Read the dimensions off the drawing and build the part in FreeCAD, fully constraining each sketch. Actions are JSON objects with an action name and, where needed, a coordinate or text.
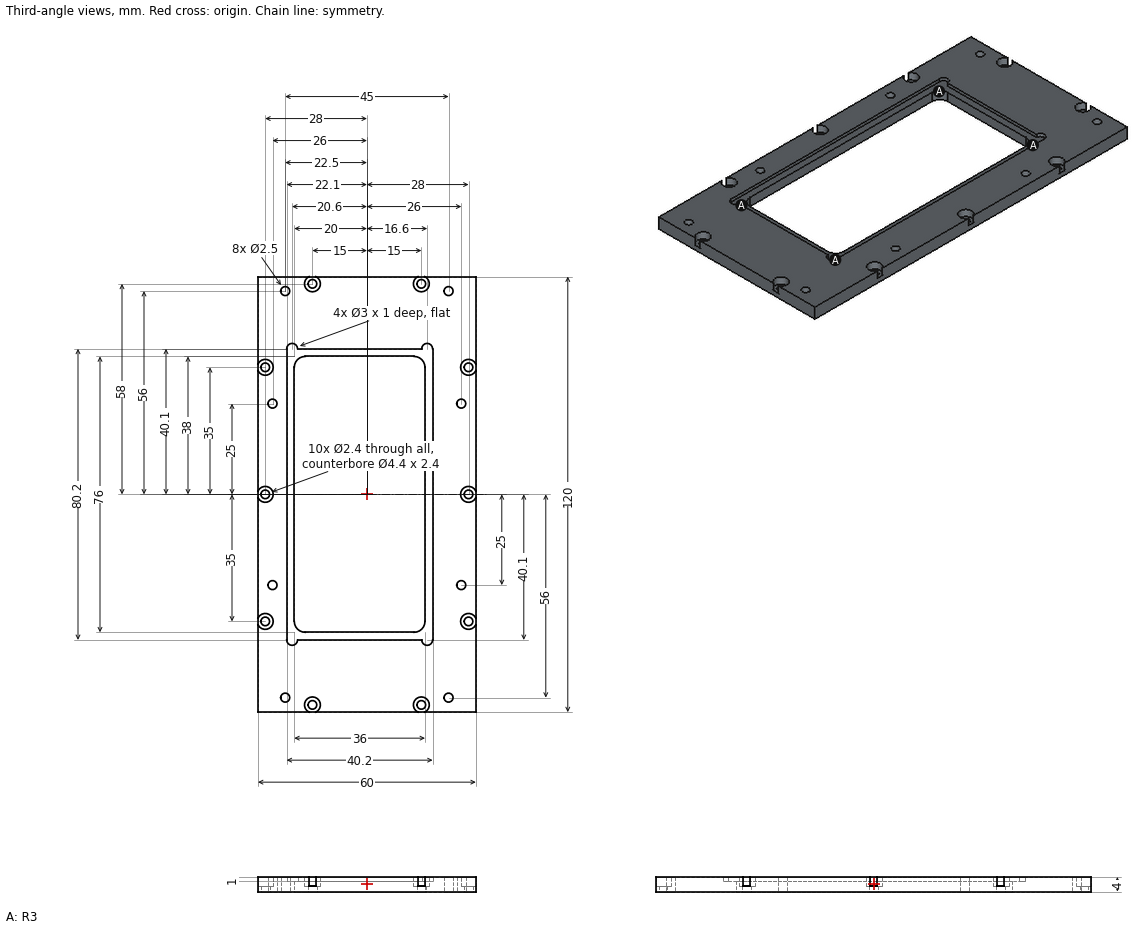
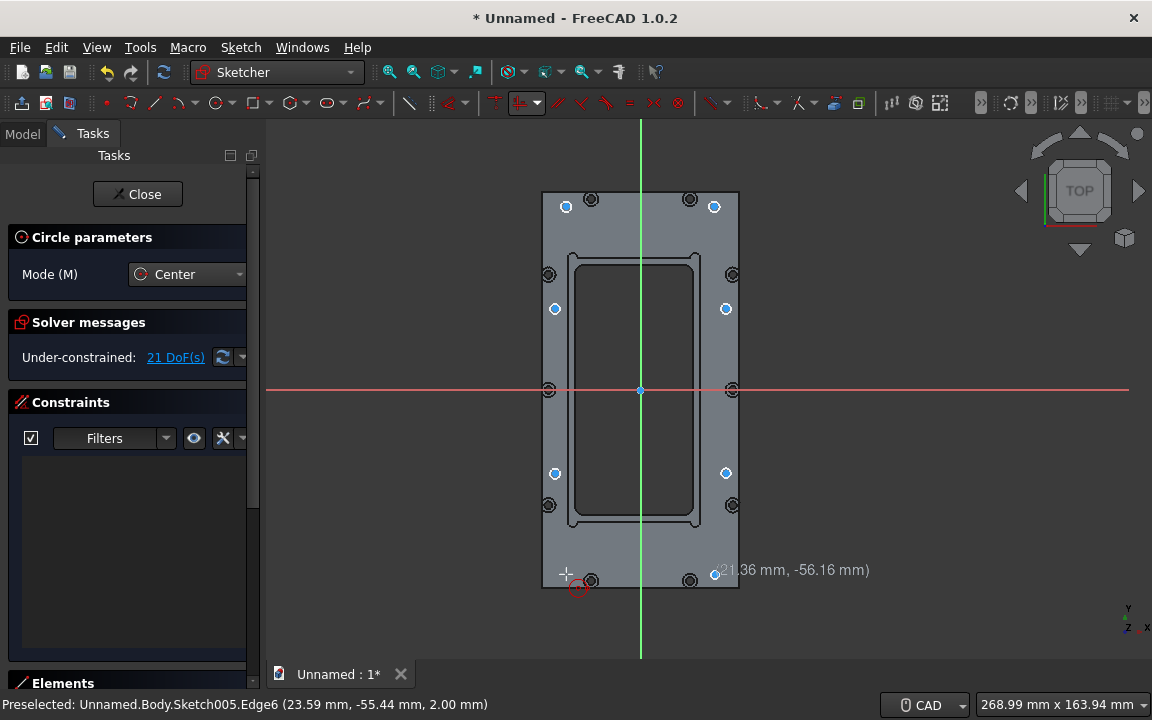
{"action": "left_click", "coordinate": [566, 574]}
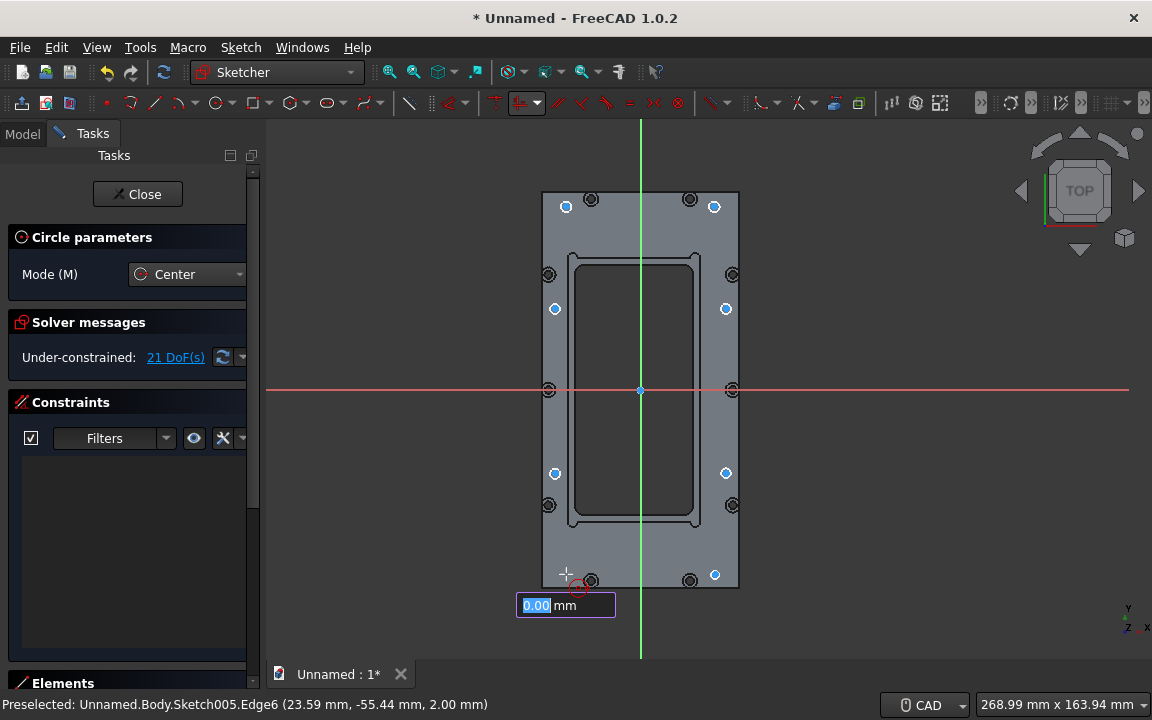
{"action": "scroll", "coordinate": [569, 572], "scroll_direction": "up", "scroll_amount": 7}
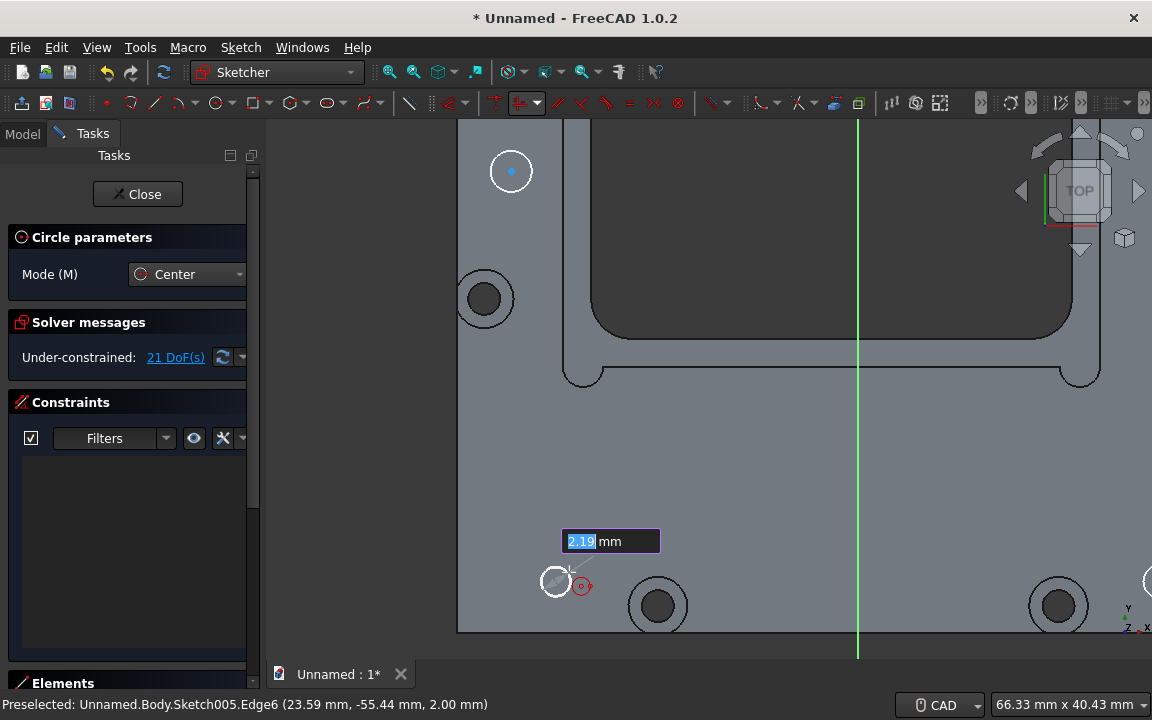
{"action": "left_click", "coordinate": [569, 568]}
{"action": "key", "text": "Escape"}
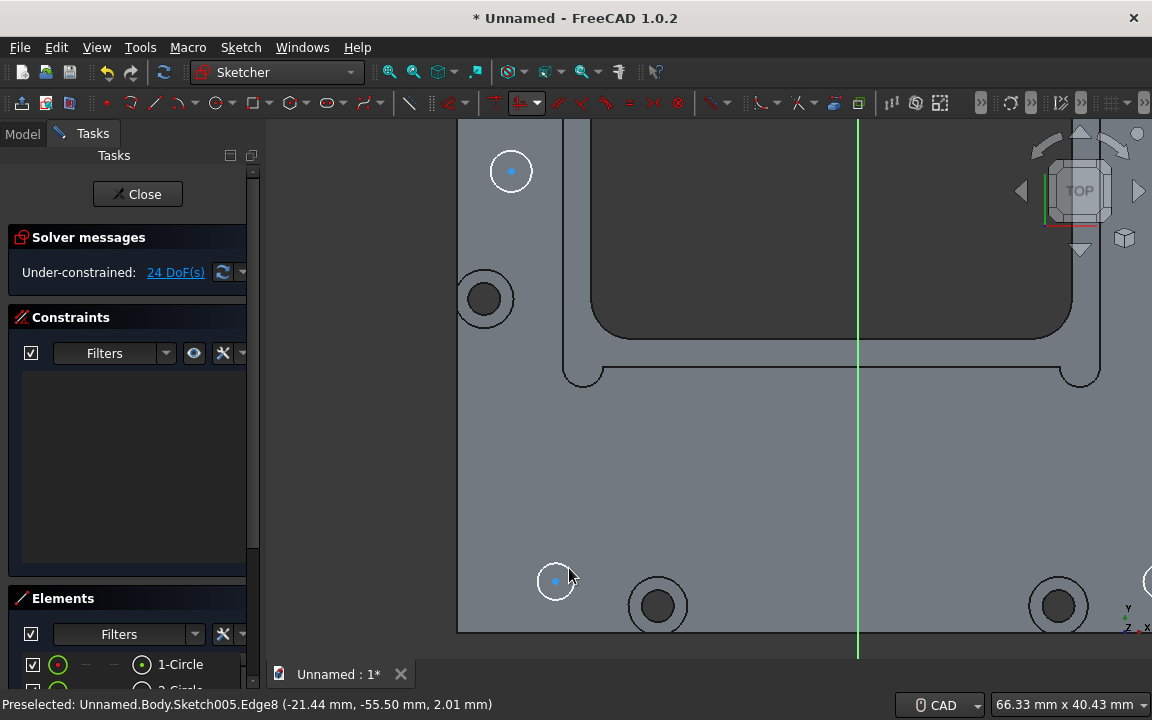
{"action": "scroll", "coordinate": [569, 572], "scroll_direction": "down", "scroll_amount": 7}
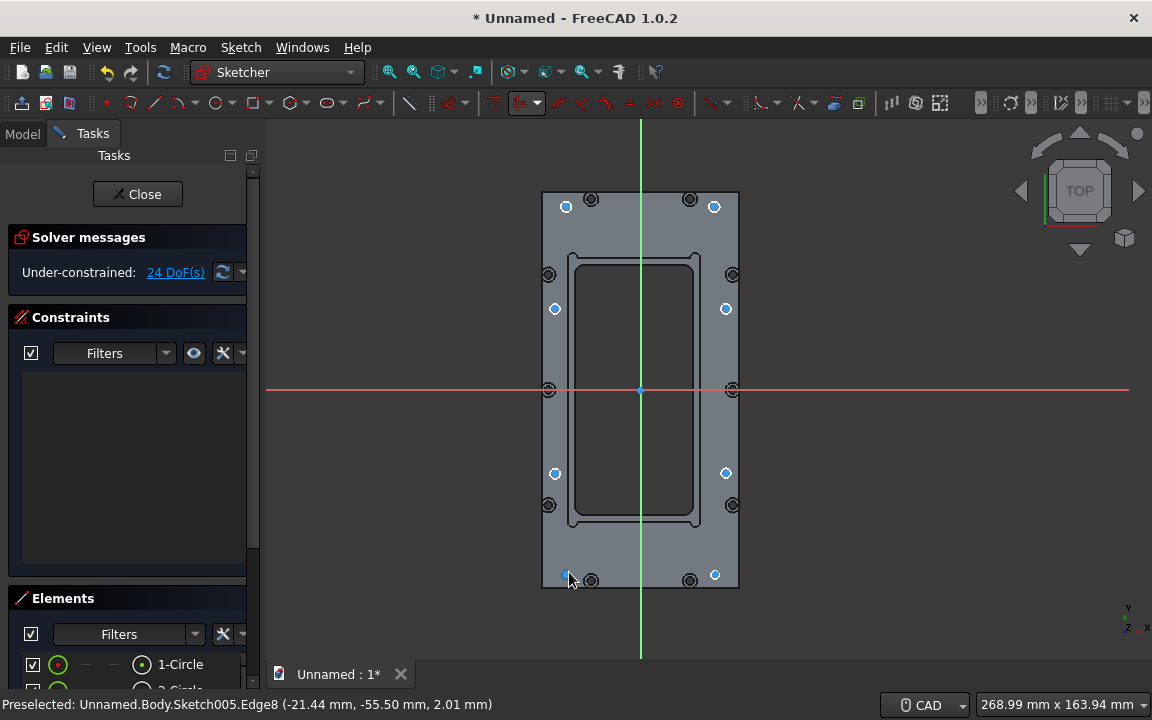
{"action": "scroll", "coordinate": [570, 203], "scroll_direction": "up", "scroll_amount": 5}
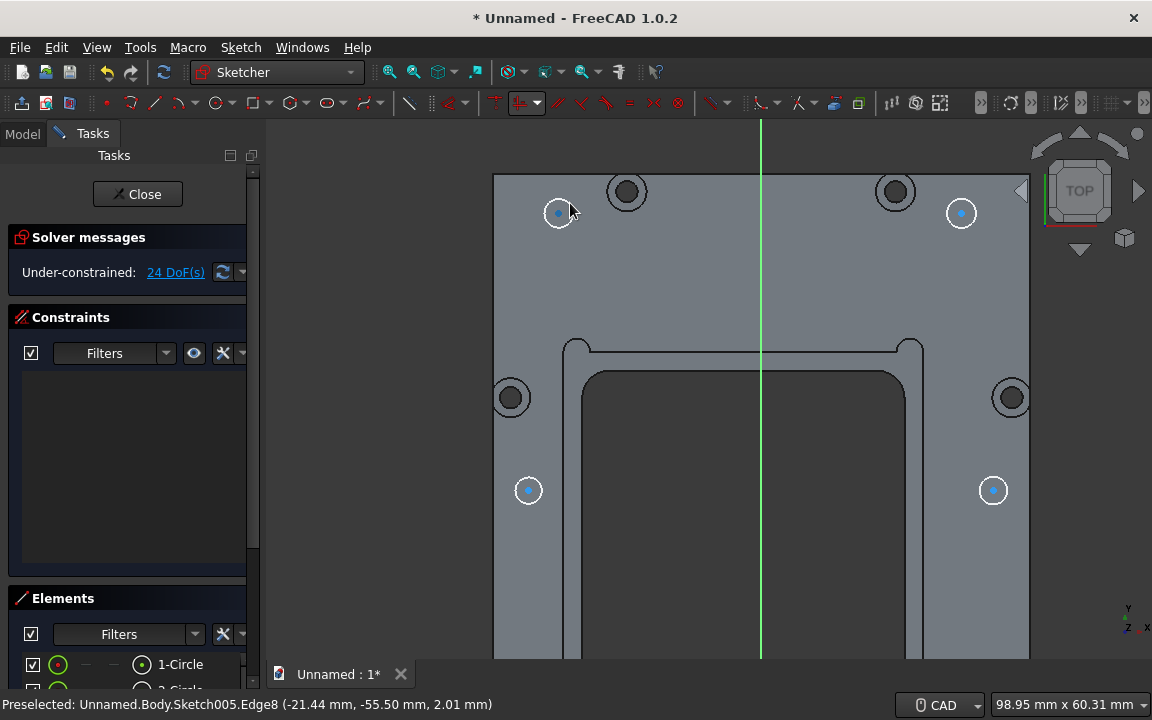
{"action": "left_click", "coordinate": [569, 203]}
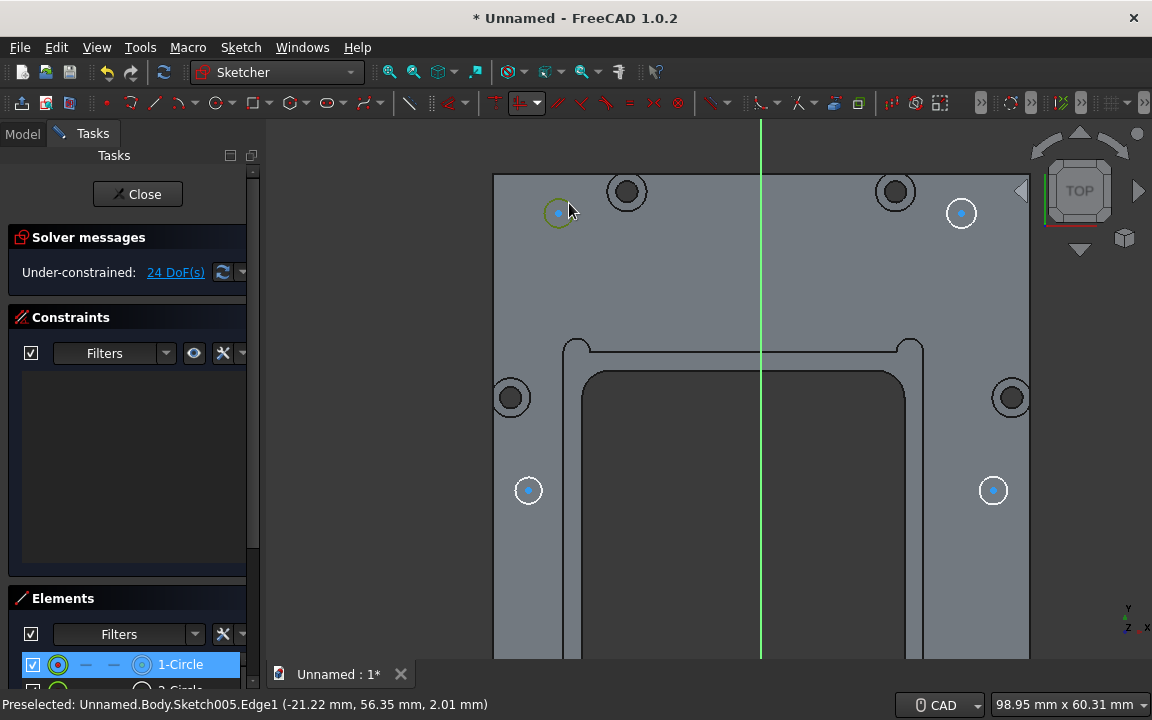
{"action": "left_click", "coordinate": [972, 203]}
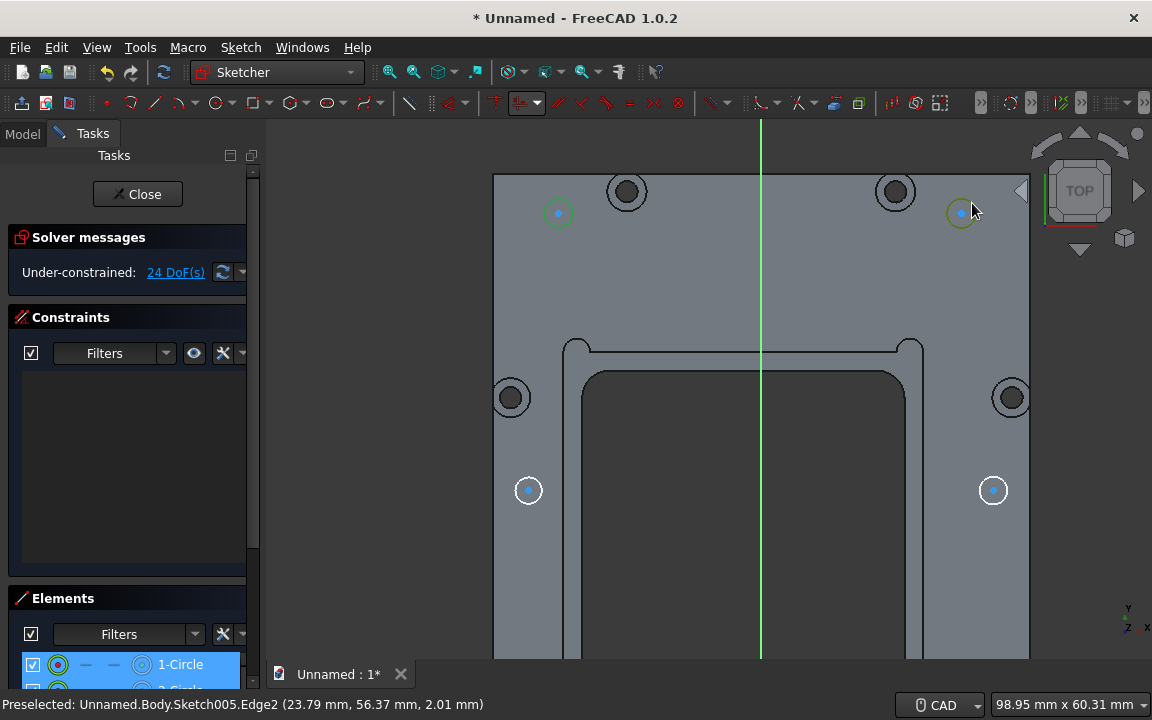
{"action": "left_click", "coordinate": [538, 481]}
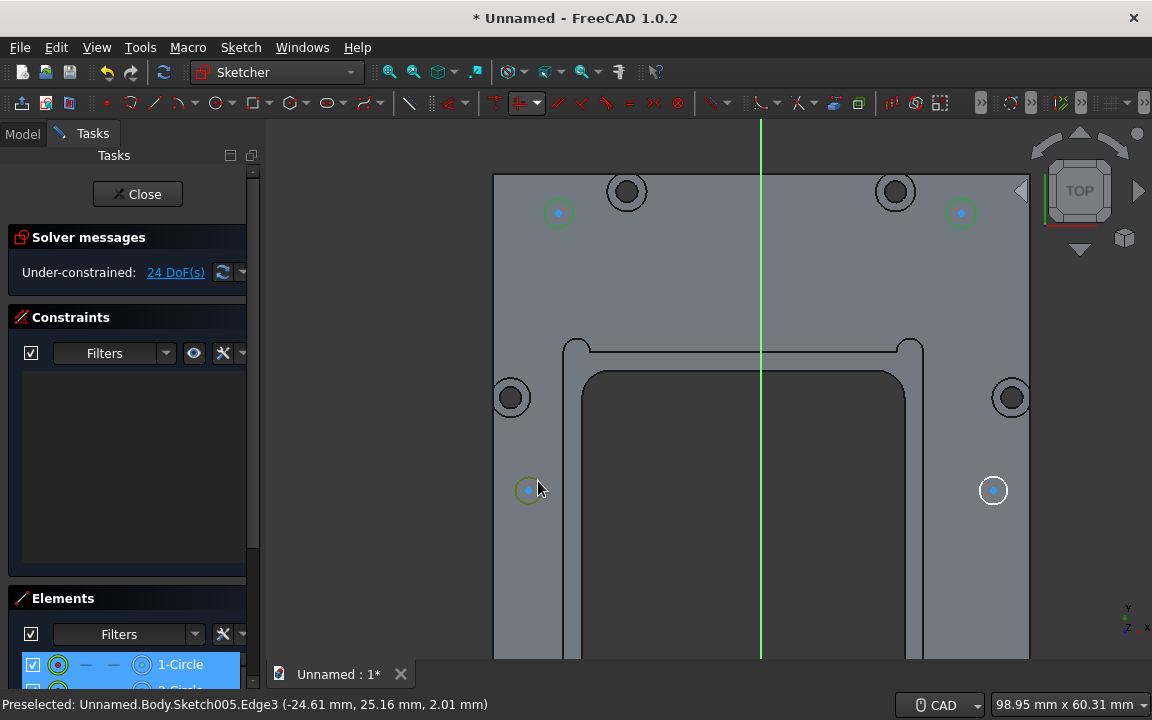
{"action": "left_click", "coordinate": [984, 481]}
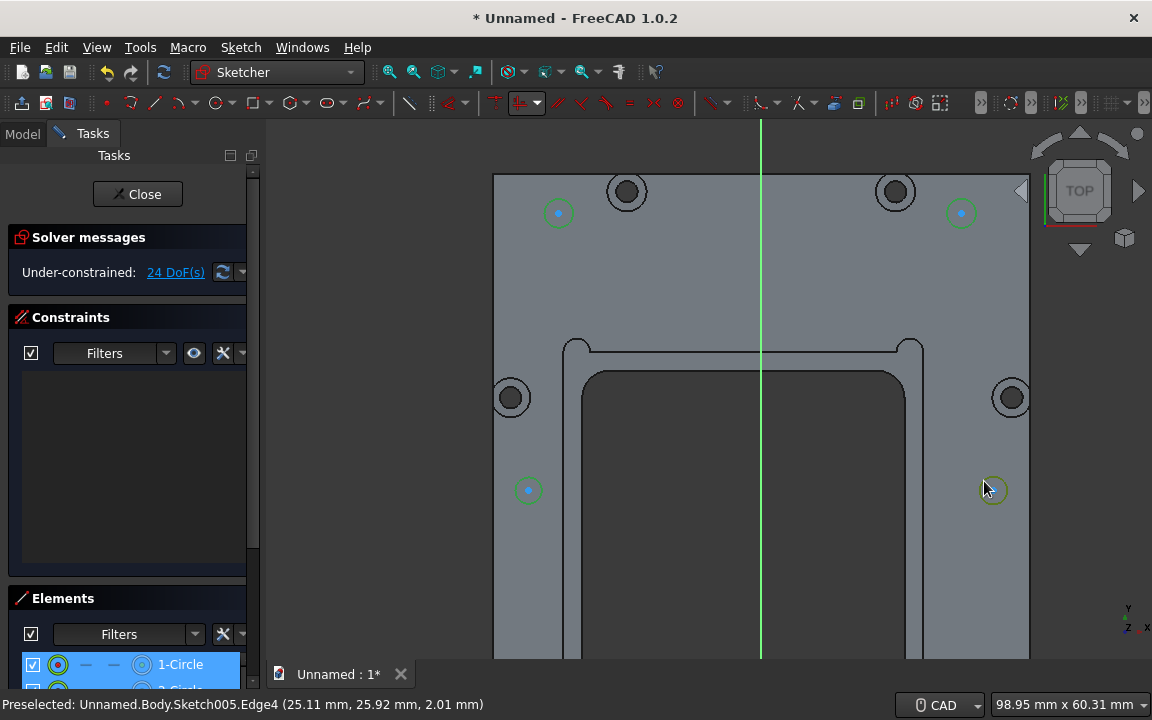
{"action": "scroll", "coordinate": [570, 202], "scroll_direction": "down", "scroll_amount": 5}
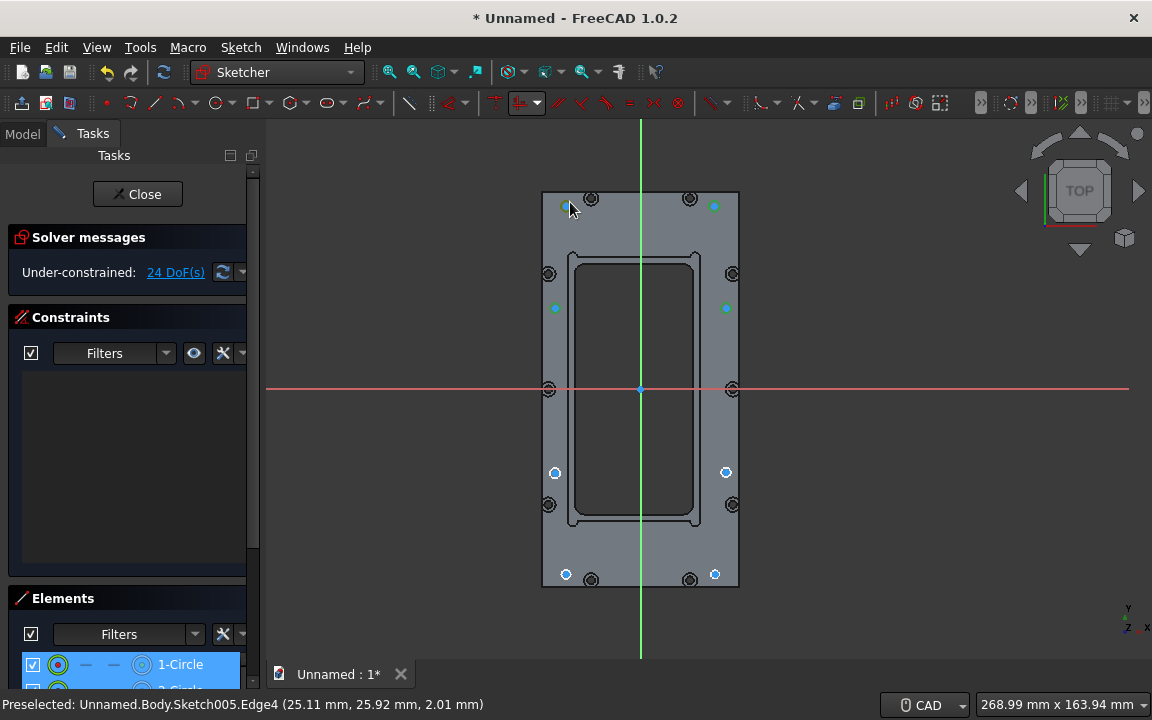
{"action": "scroll", "coordinate": [729, 469], "scroll_direction": "up", "scroll_amount": 6}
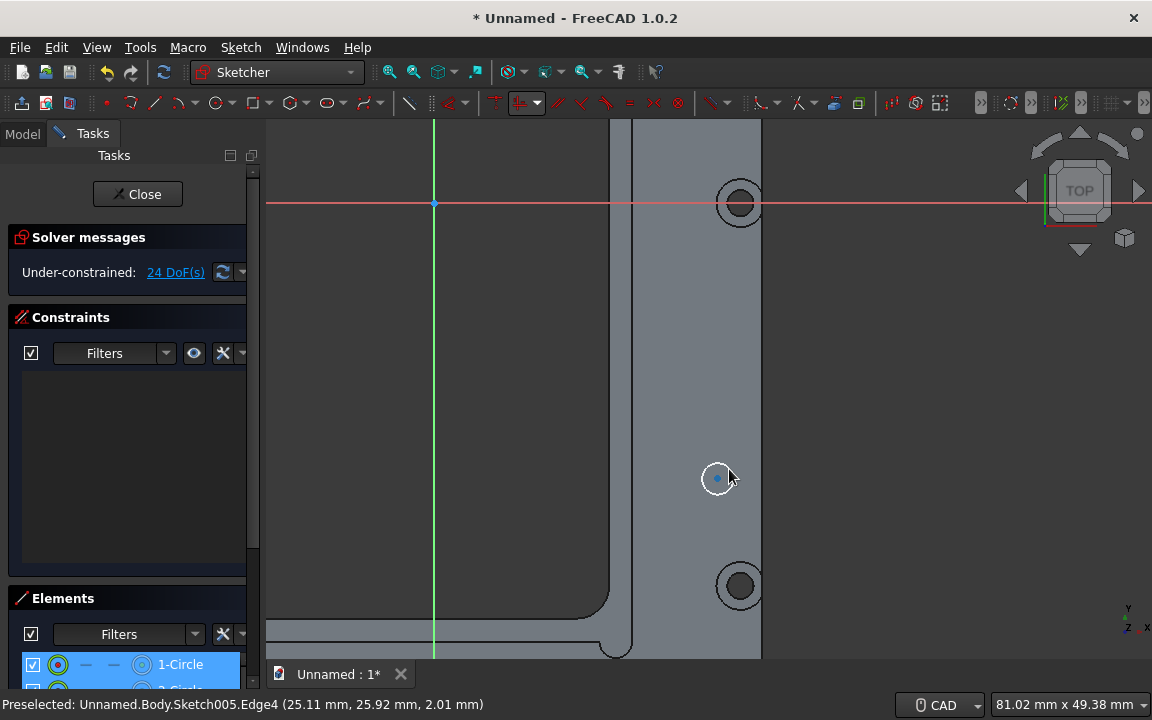
{"action": "left_click", "coordinate": [729, 468]}